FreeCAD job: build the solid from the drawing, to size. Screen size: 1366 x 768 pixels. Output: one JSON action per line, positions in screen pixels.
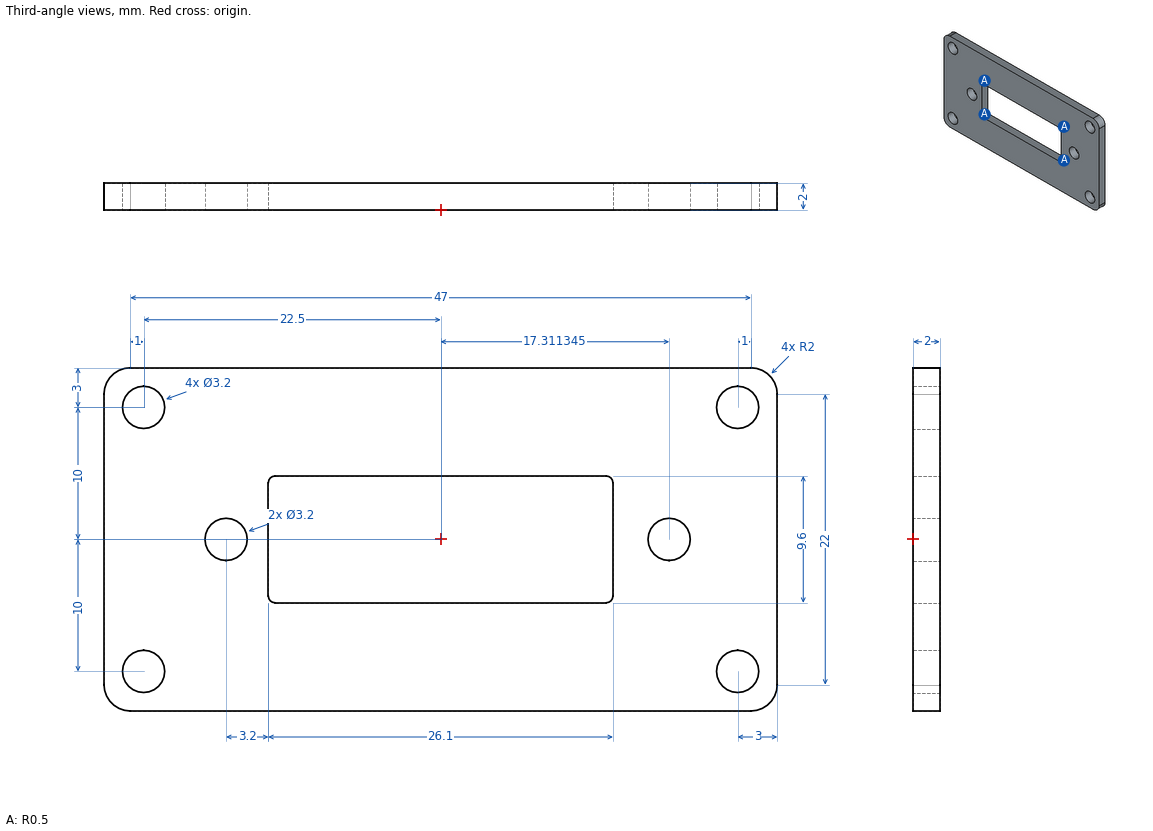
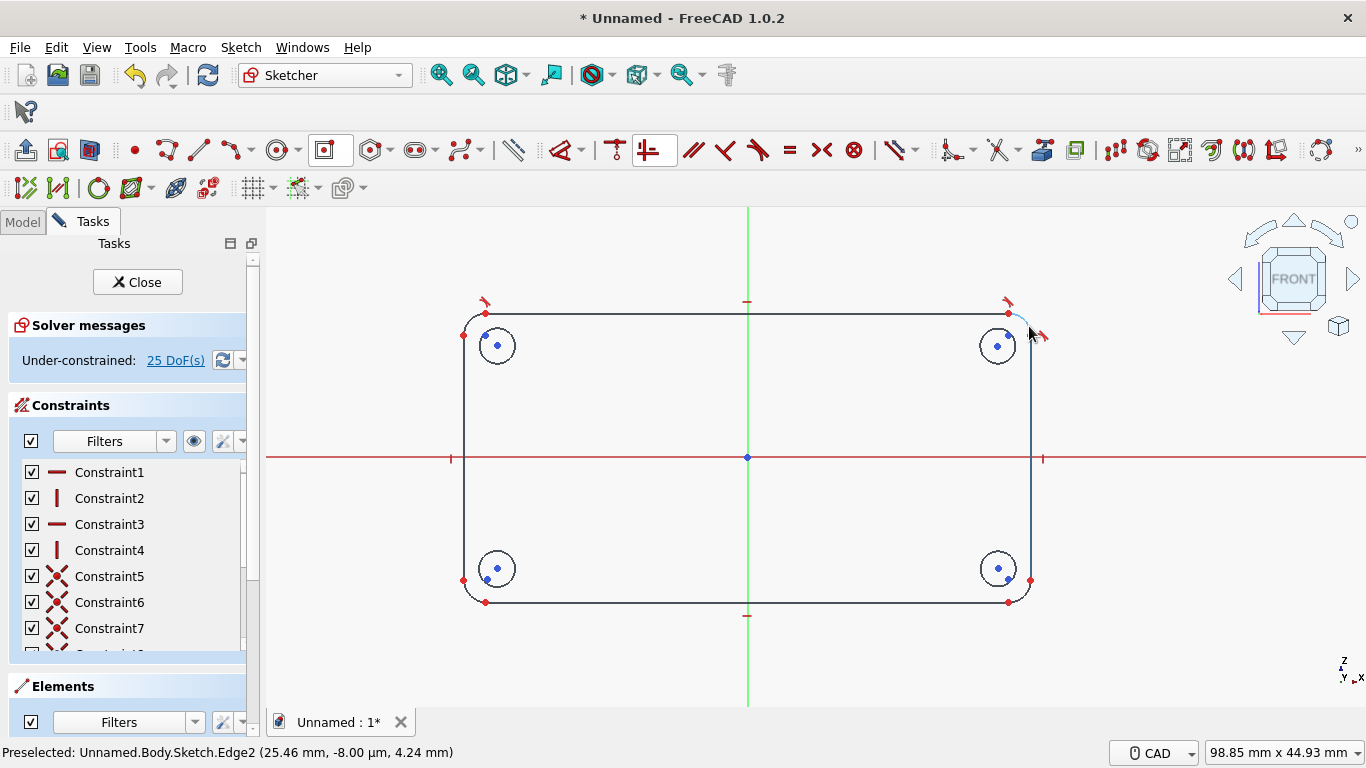
{"action": "scroll", "coordinate": [1019, 600], "scroll_direction": "up", "scroll_amount": 2}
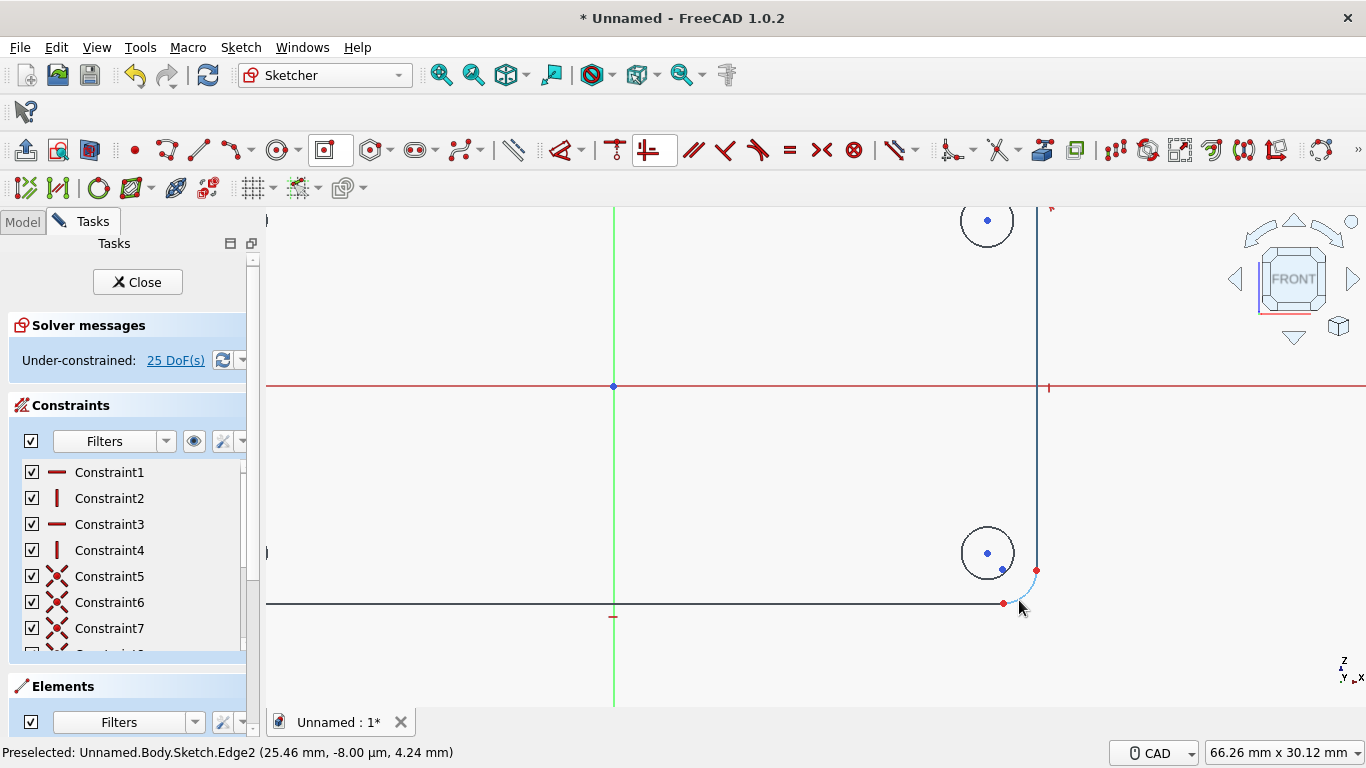
{"action": "left_click", "coordinate": [1018, 600]}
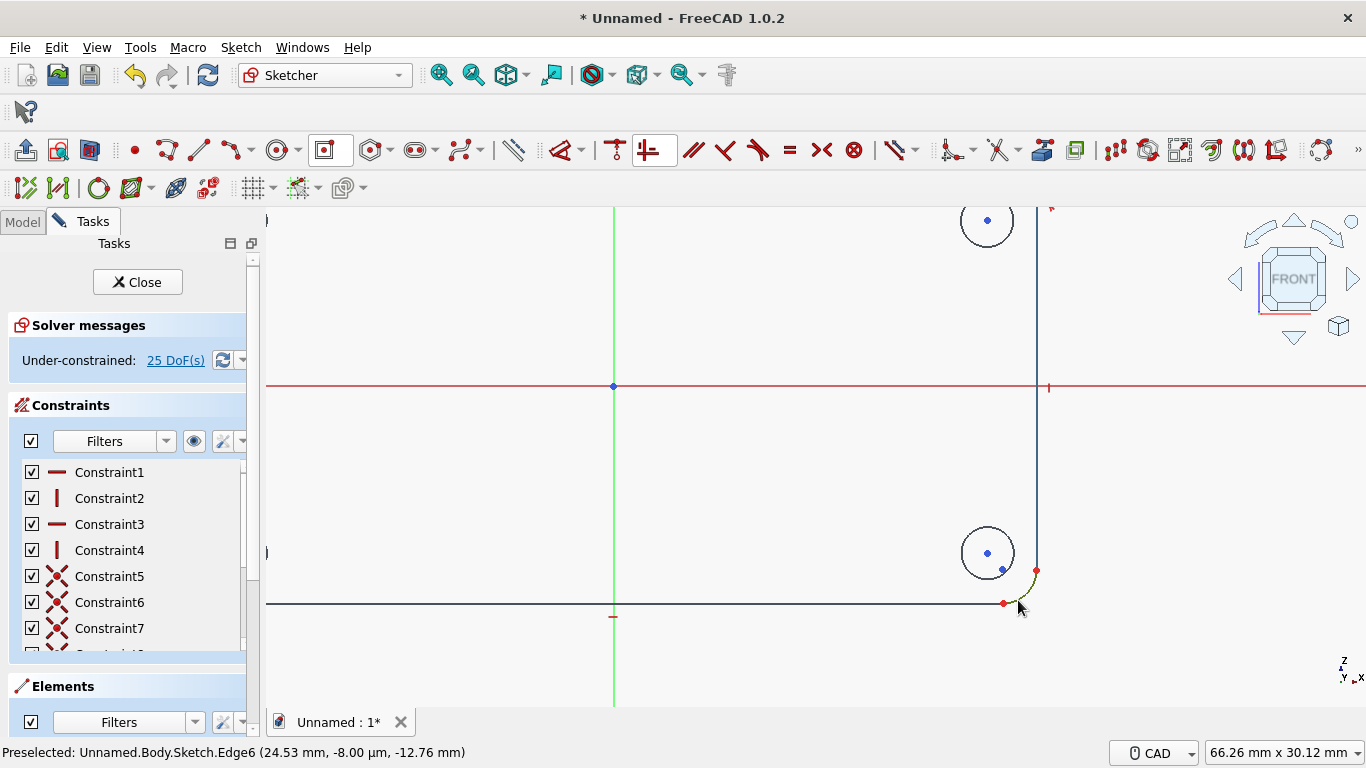
{"action": "left_click", "coordinate": [758, 150]}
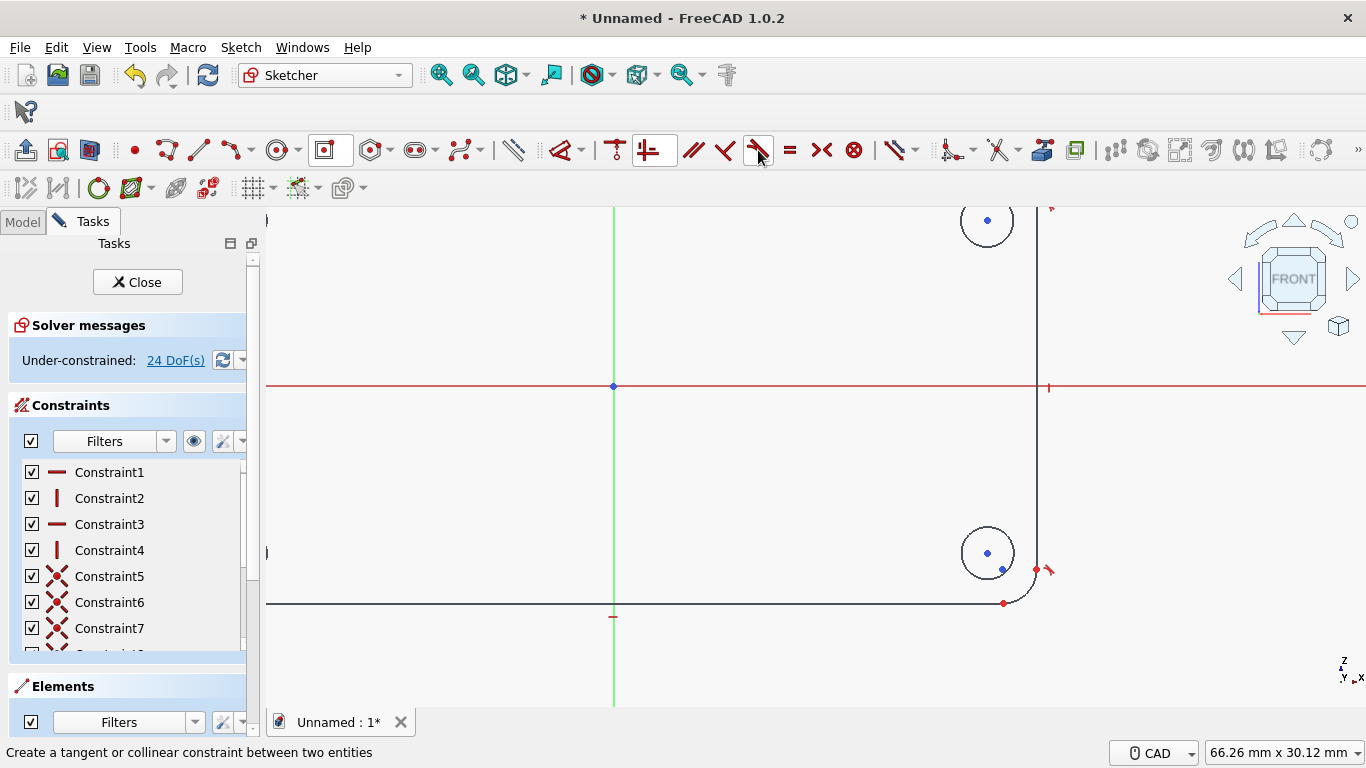
{"action": "left_click", "coordinate": [770, 604]}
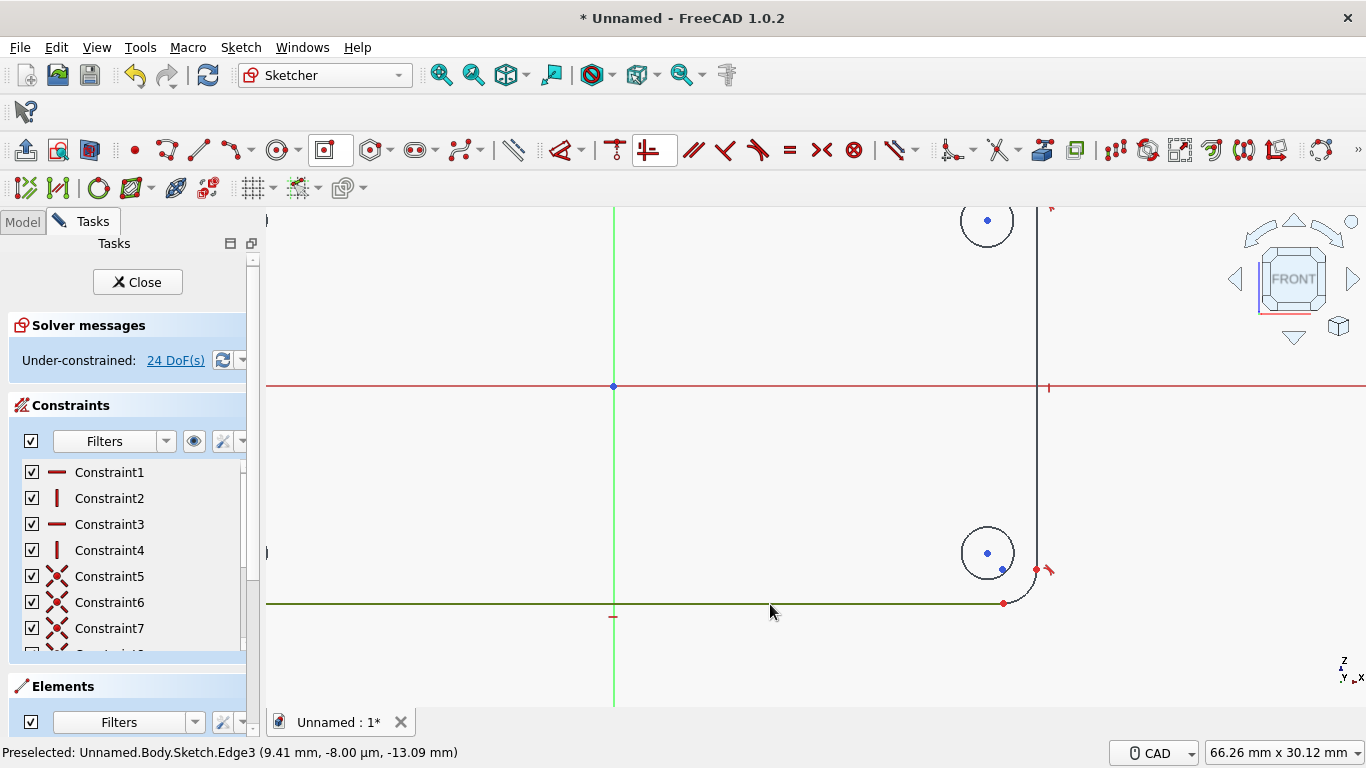
{"action": "left_click", "coordinate": [1019, 599]}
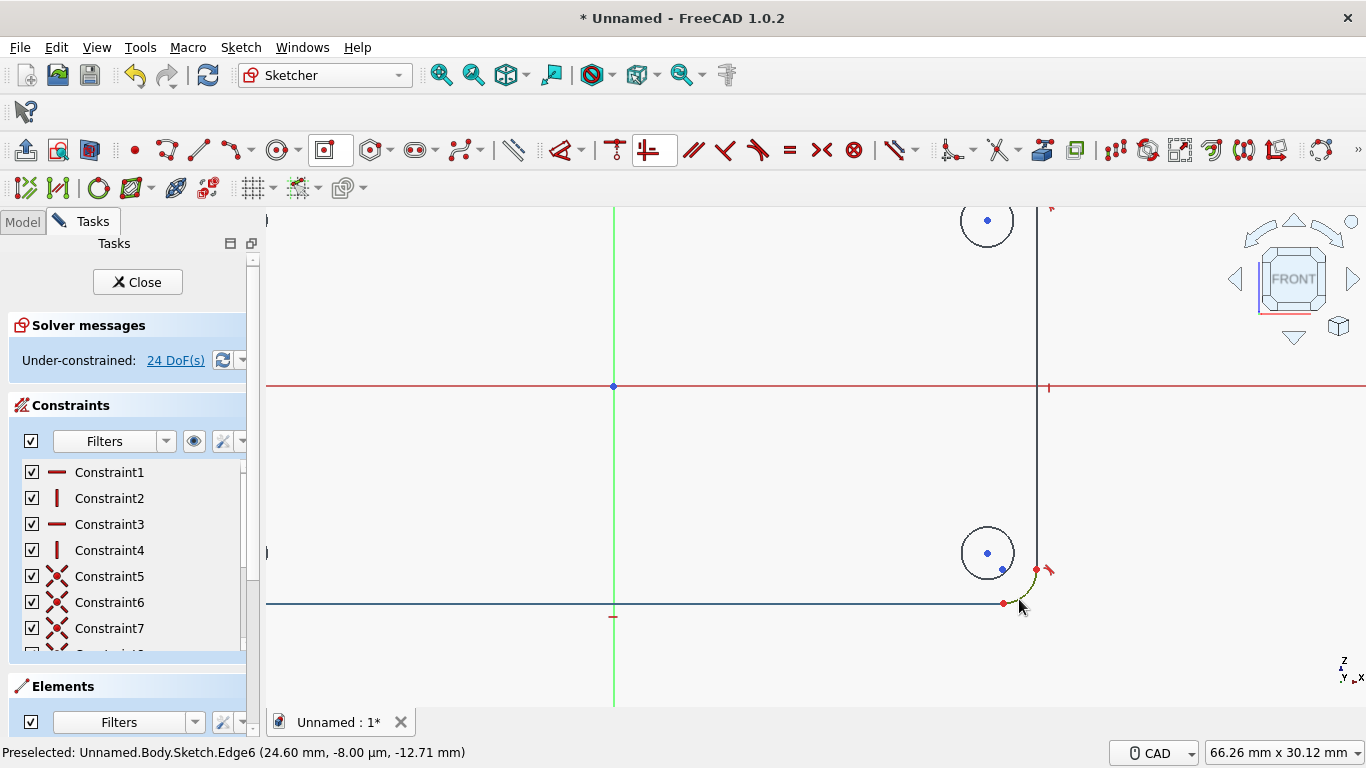
{"action": "left_click", "coordinate": [758, 150]}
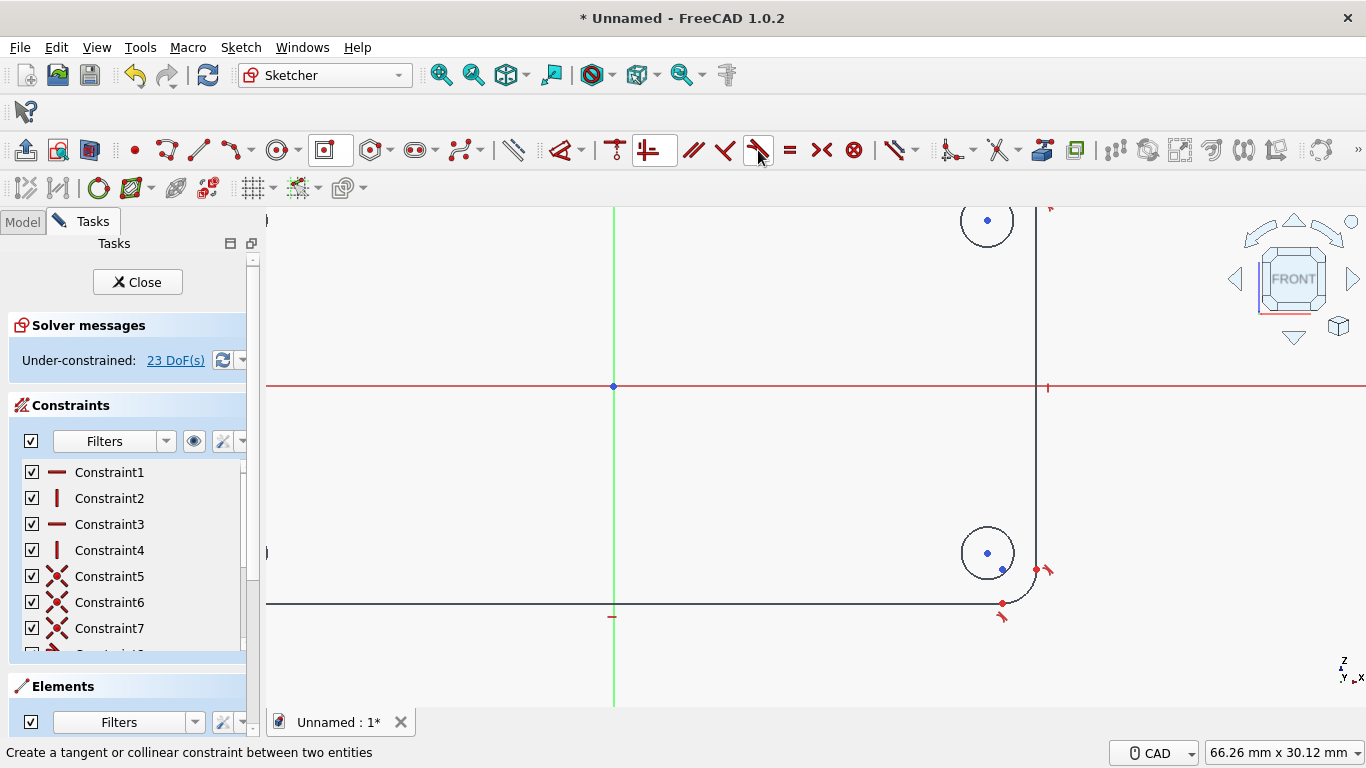
{"action": "left_click", "coordinate": [769, 604]}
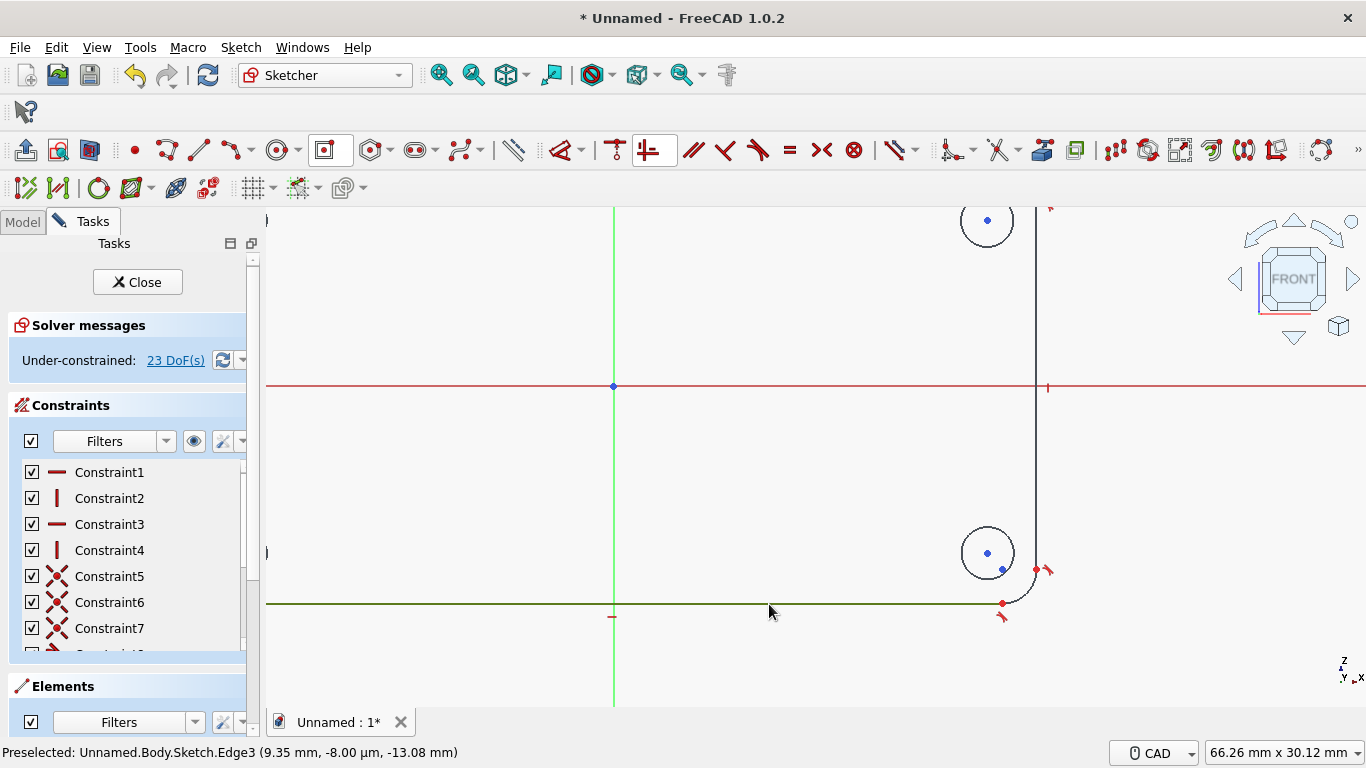
{"action": "scroll", "coordinate": [1019, 601], "scroll_direction": "down", "scroll_amount": 2}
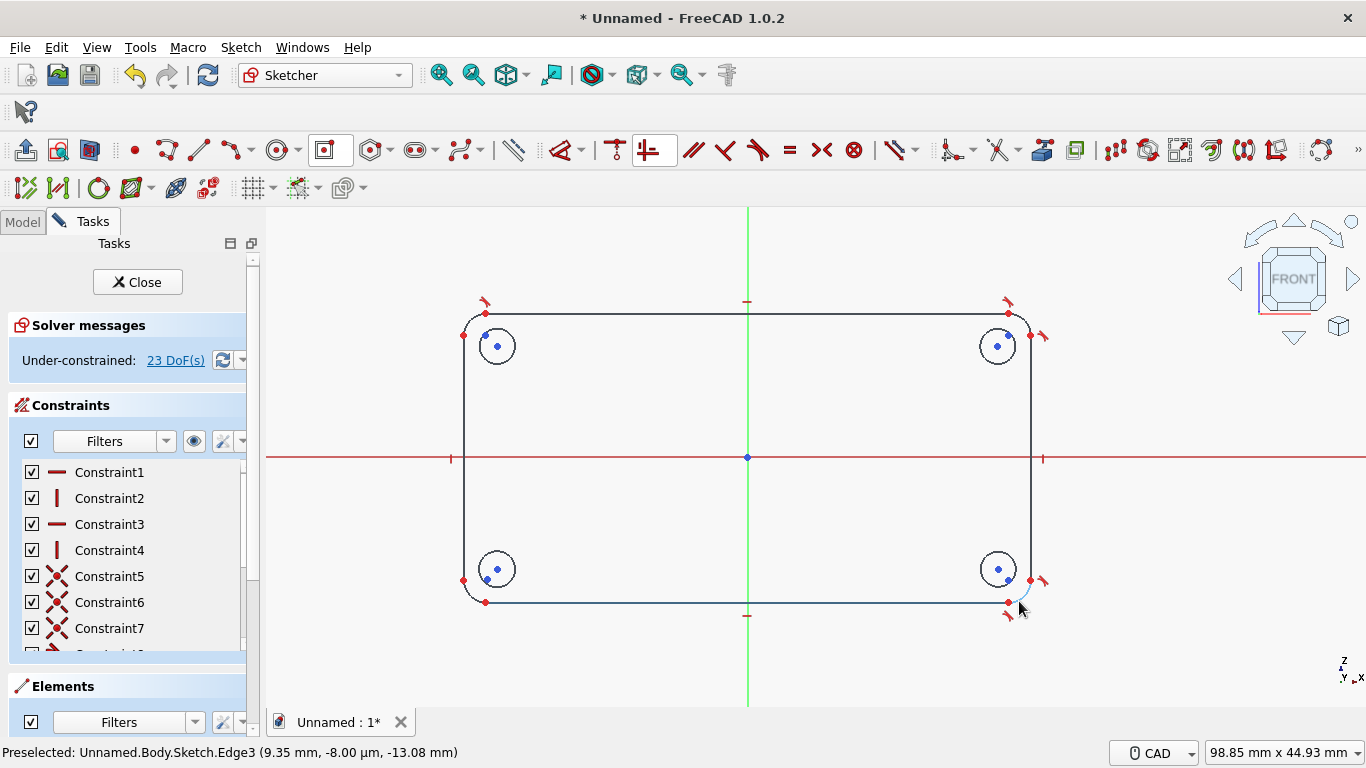
{"action": "scroll", "coordinate": [467, 591], "scroll_direction": "up", "scroll_amount": 2}